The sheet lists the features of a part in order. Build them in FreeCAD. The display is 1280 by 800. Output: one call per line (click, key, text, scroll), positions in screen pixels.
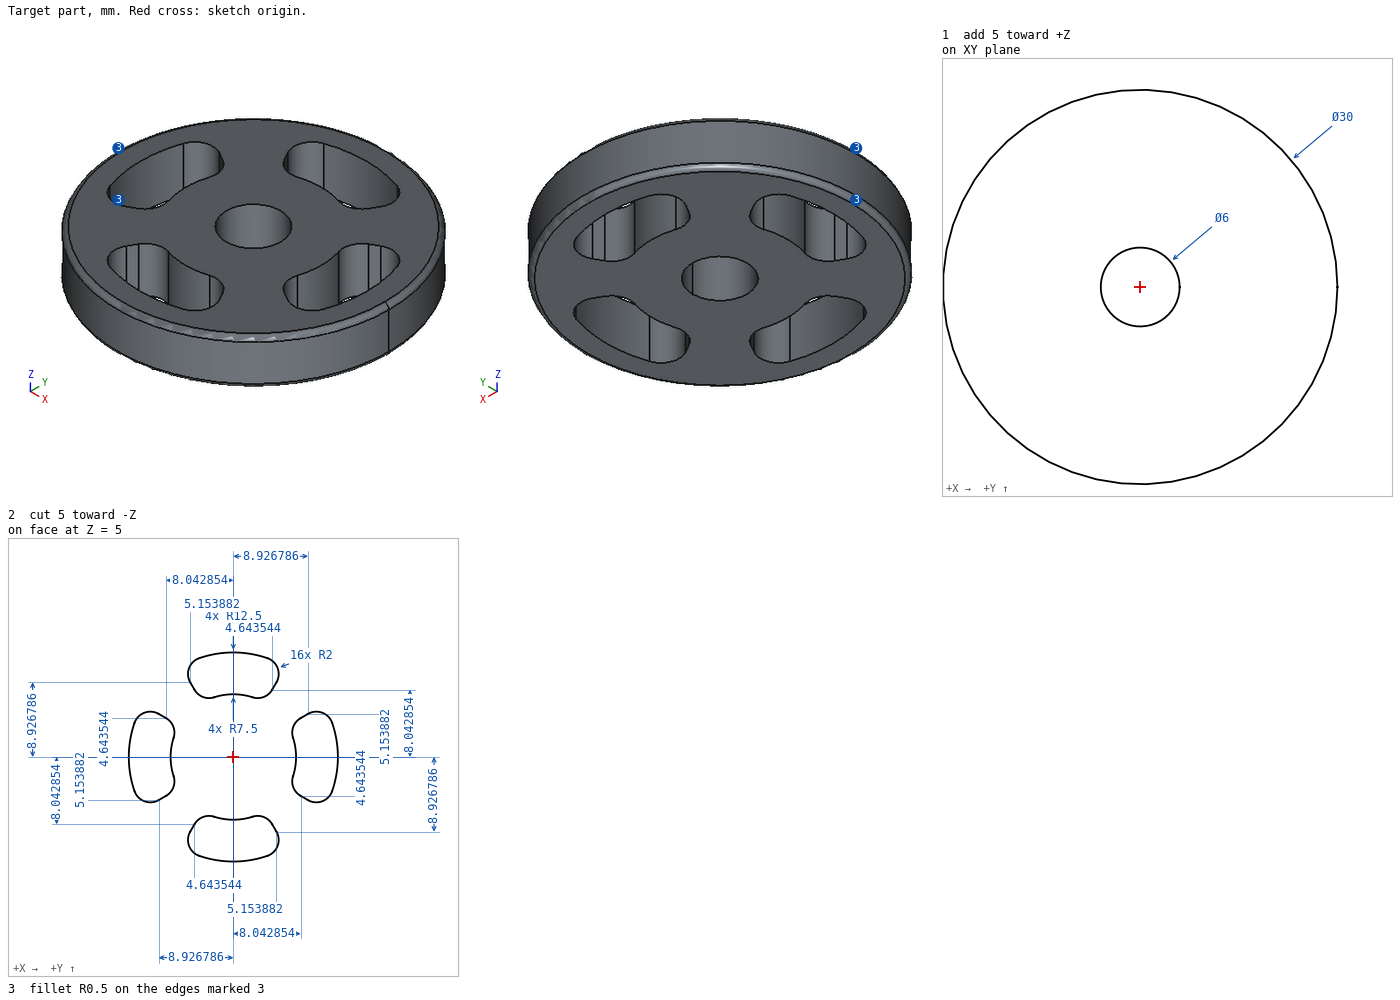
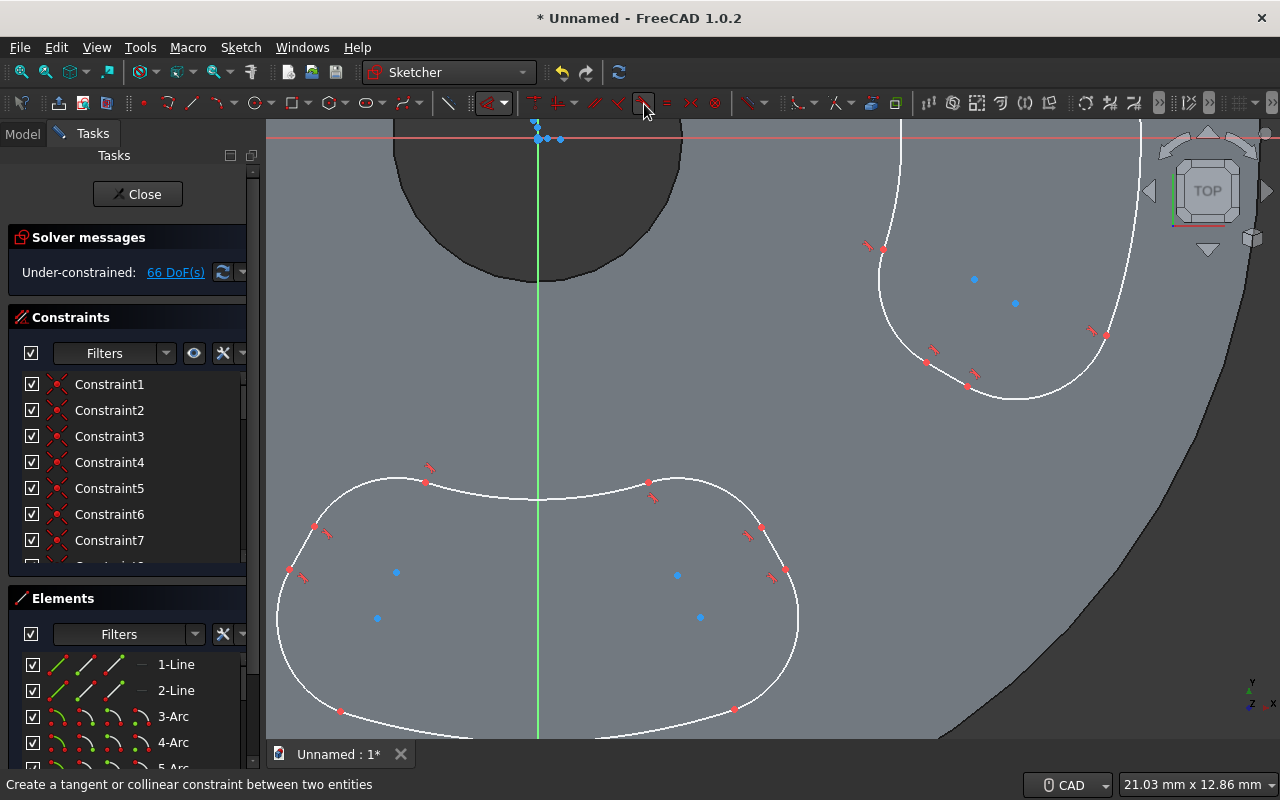
click(299, 682)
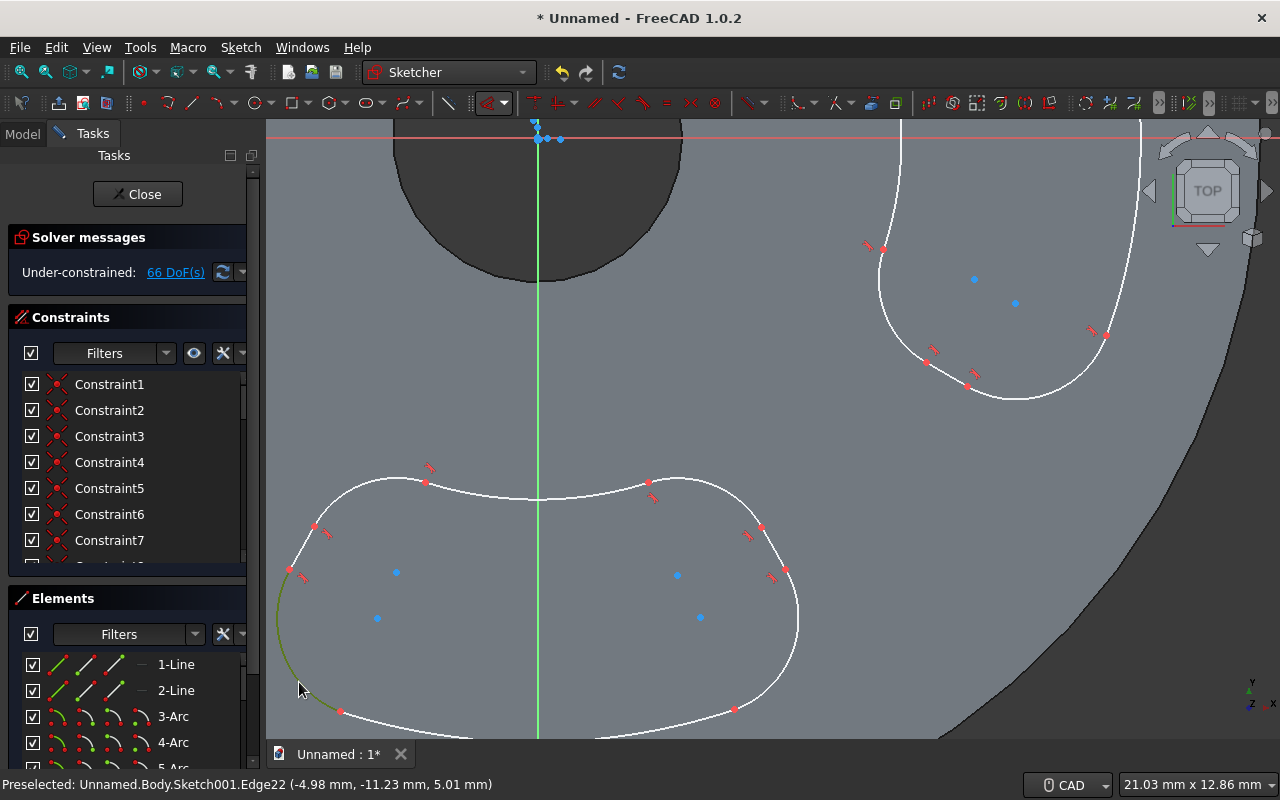
scroll(776, 555, down, 6)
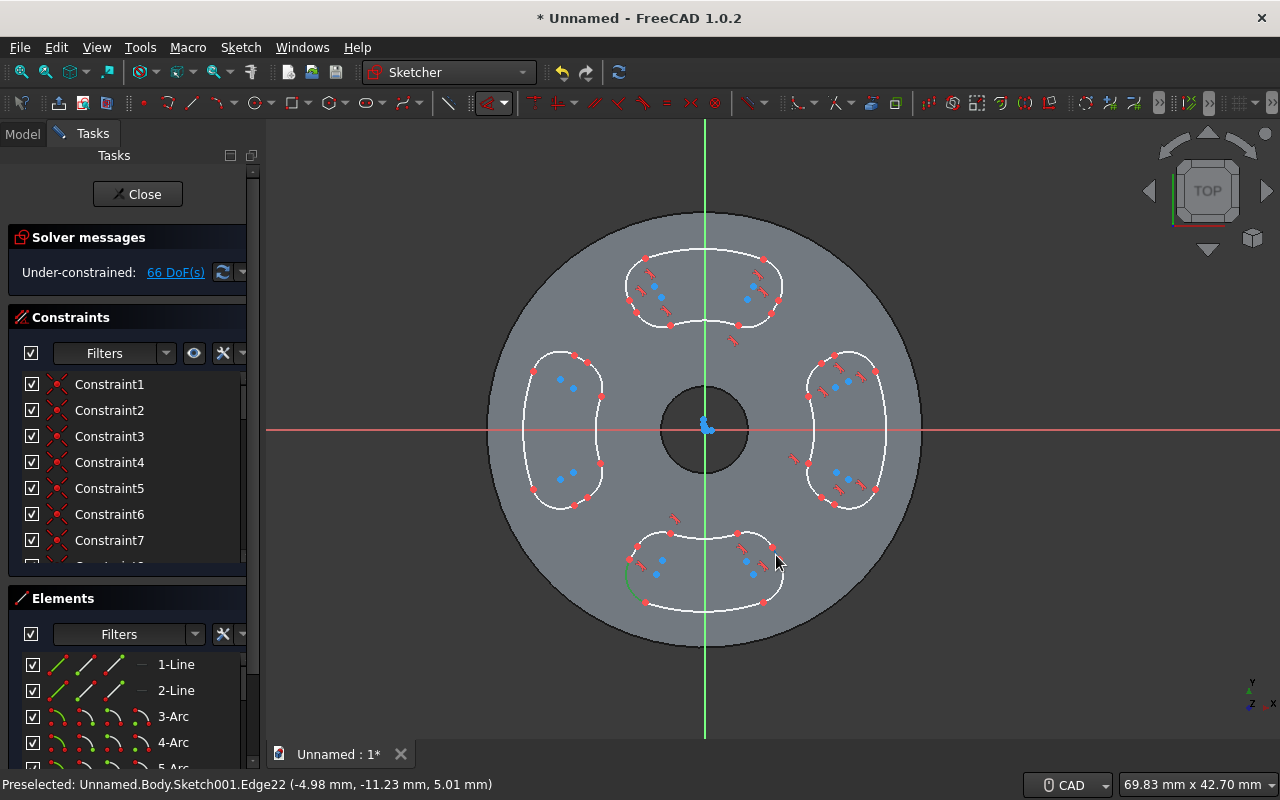
click(680, 610)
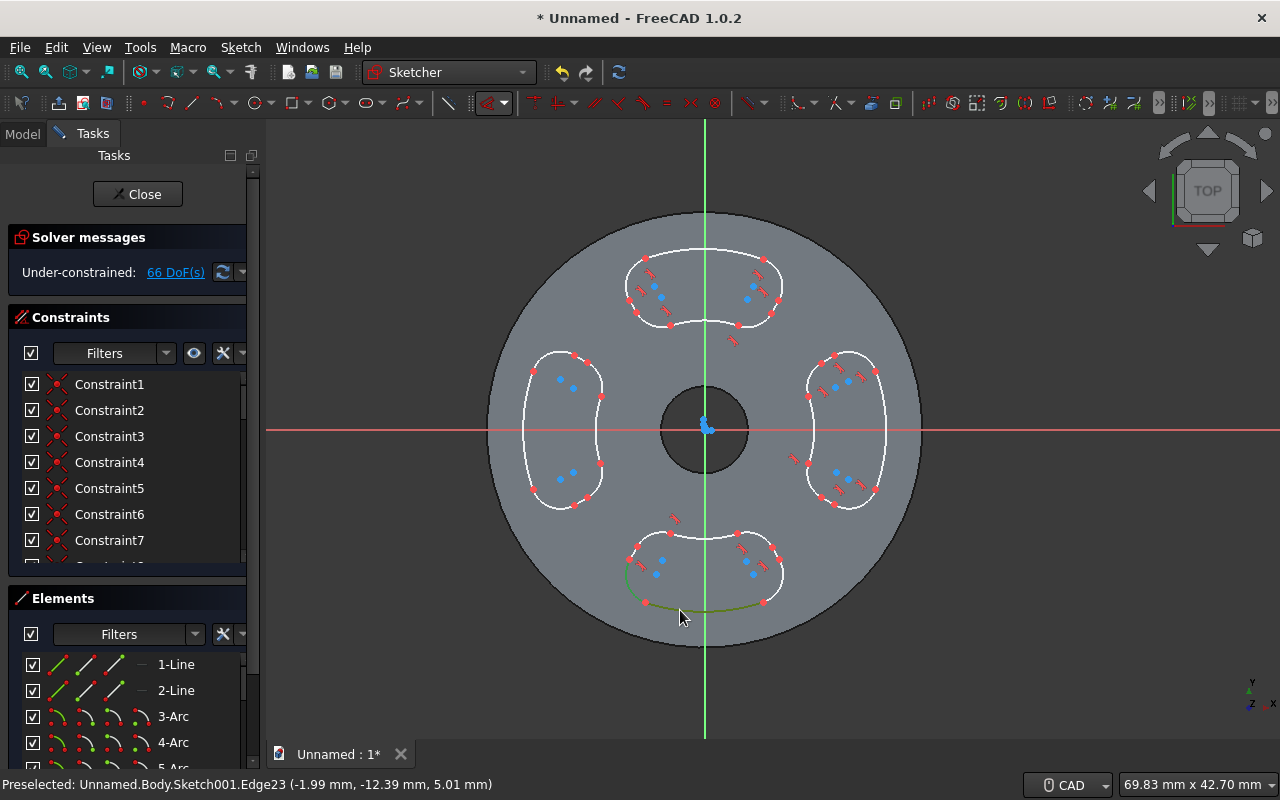
click(644, 104)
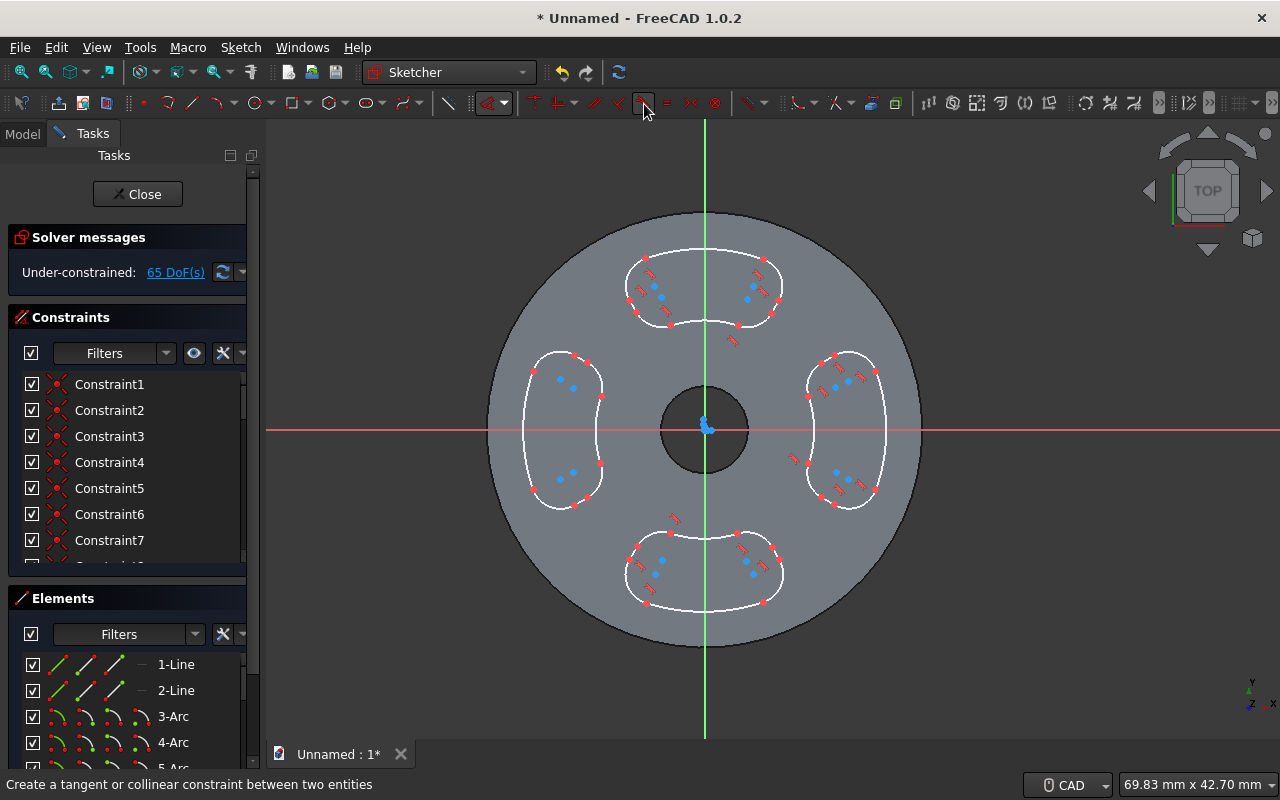
click(681, 610)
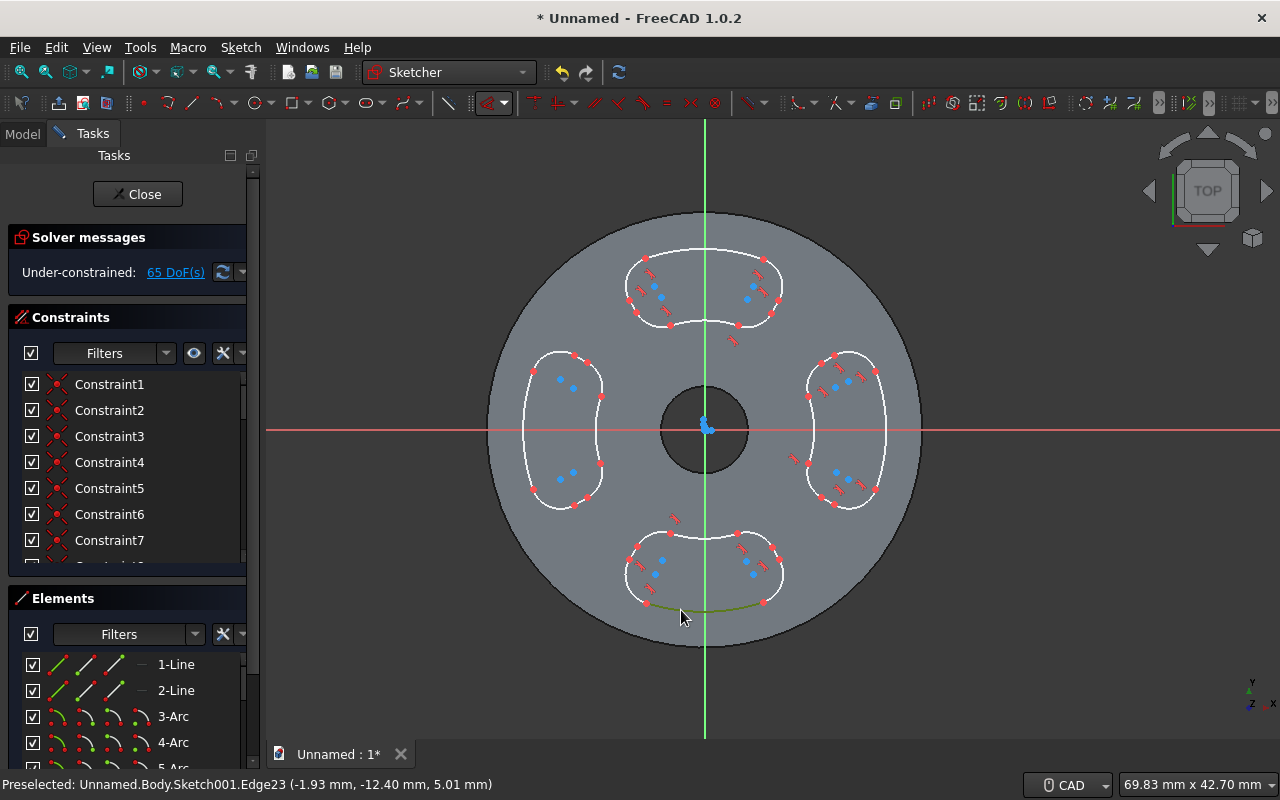
click(776, 593)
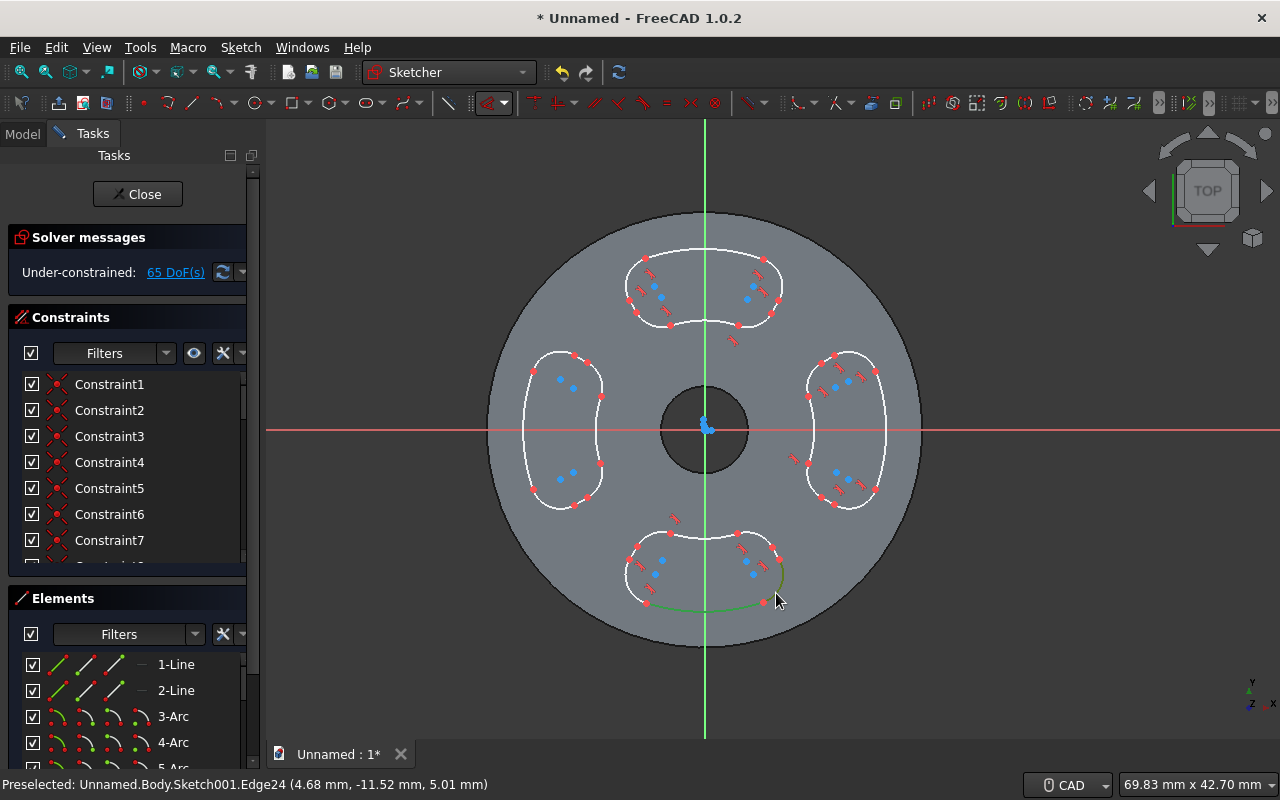
click(644, 104)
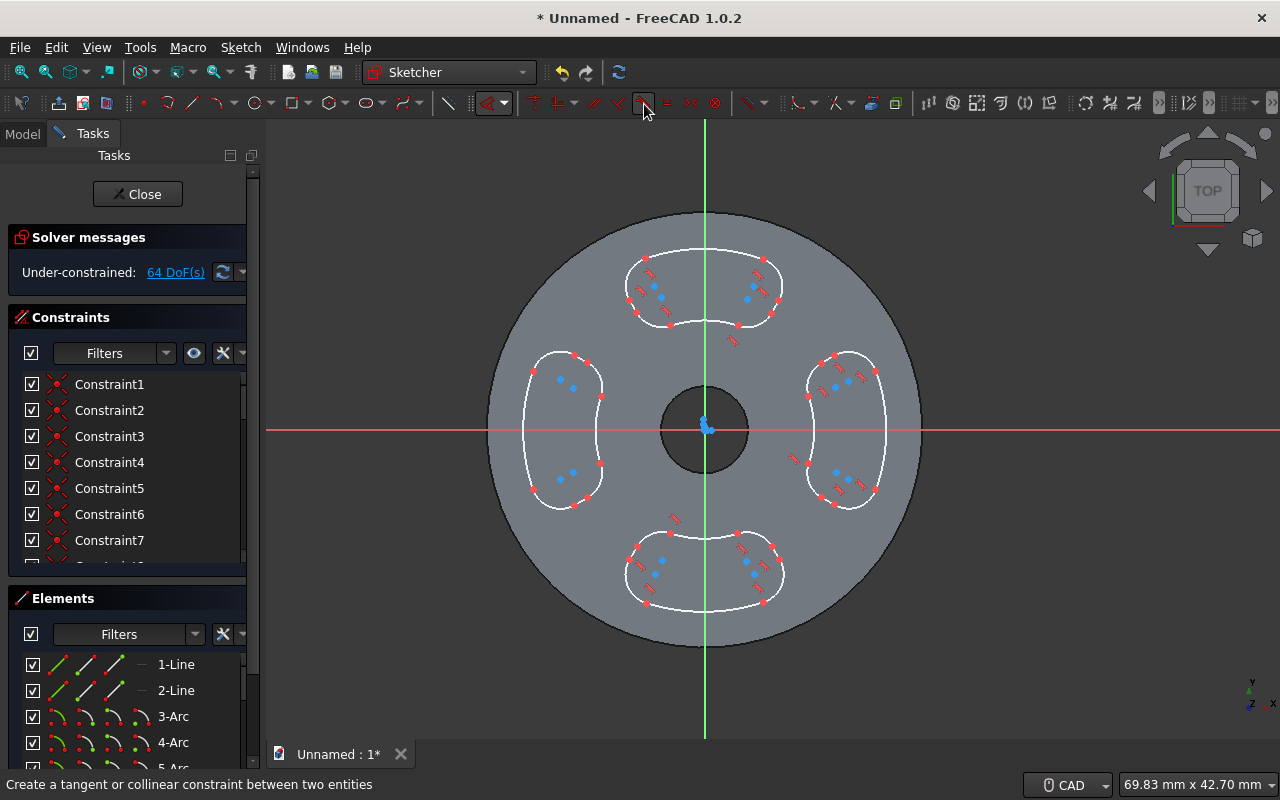
scroll(581, 501, up, 4)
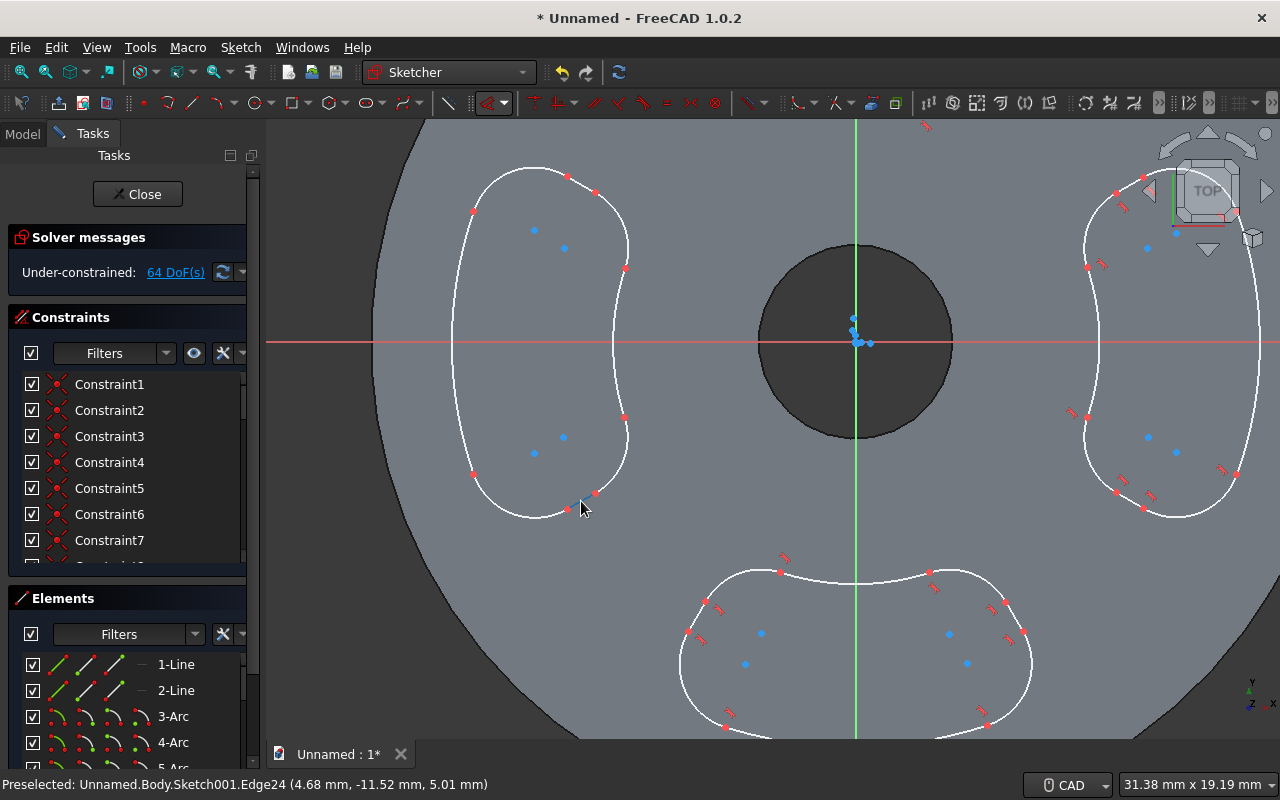
click(581, 501)